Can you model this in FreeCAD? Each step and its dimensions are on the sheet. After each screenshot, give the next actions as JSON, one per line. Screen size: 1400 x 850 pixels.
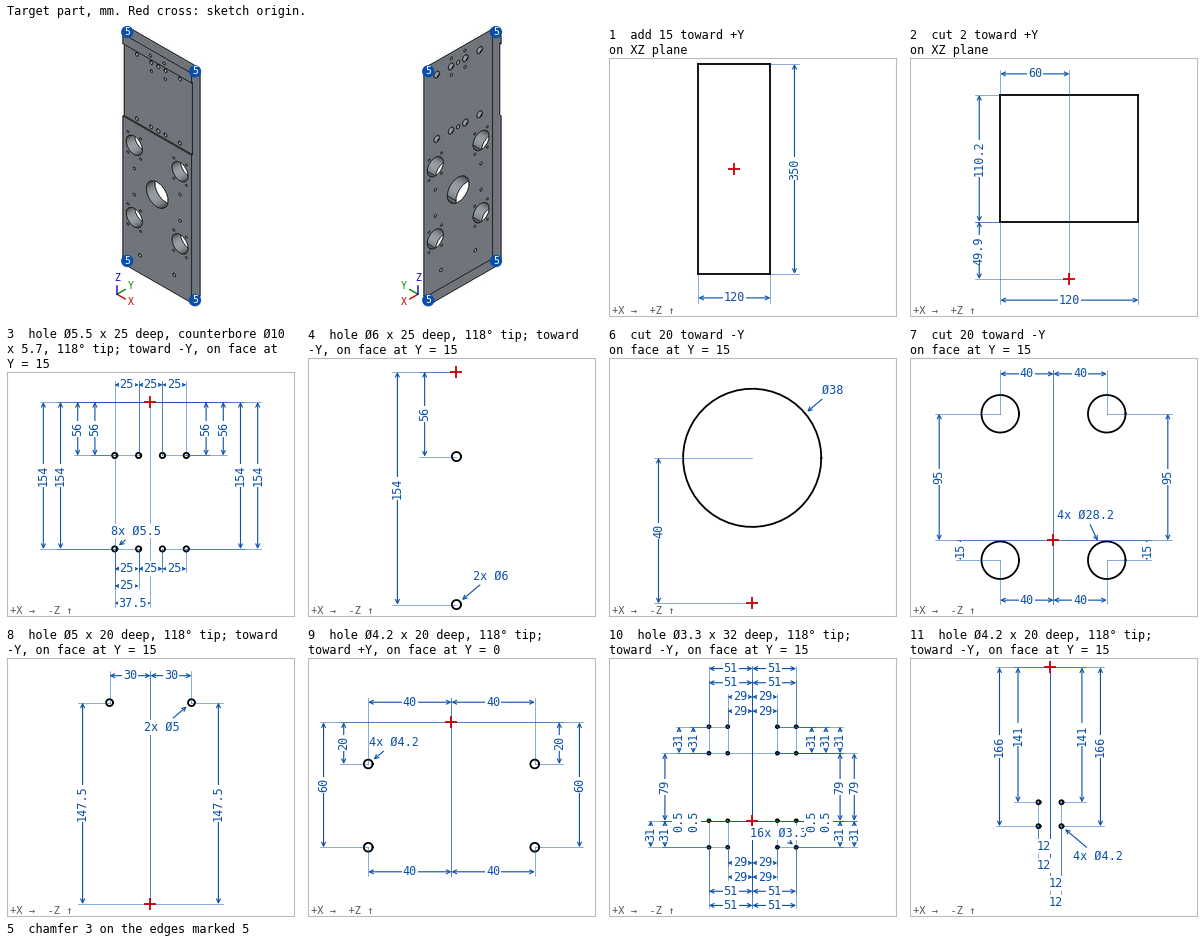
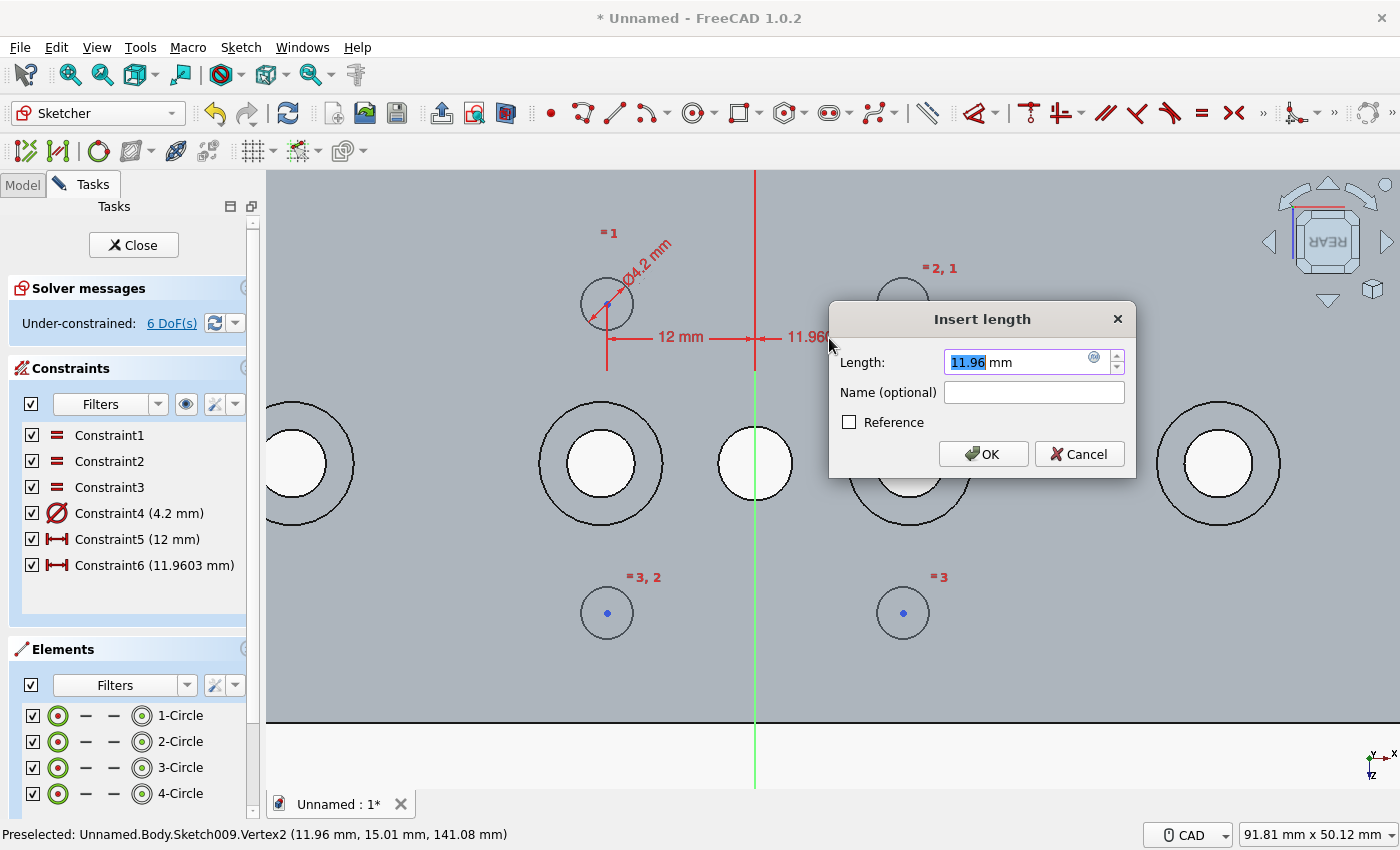
{"action": "type", "text": "12"}
{"action": "key", "text": "Return"}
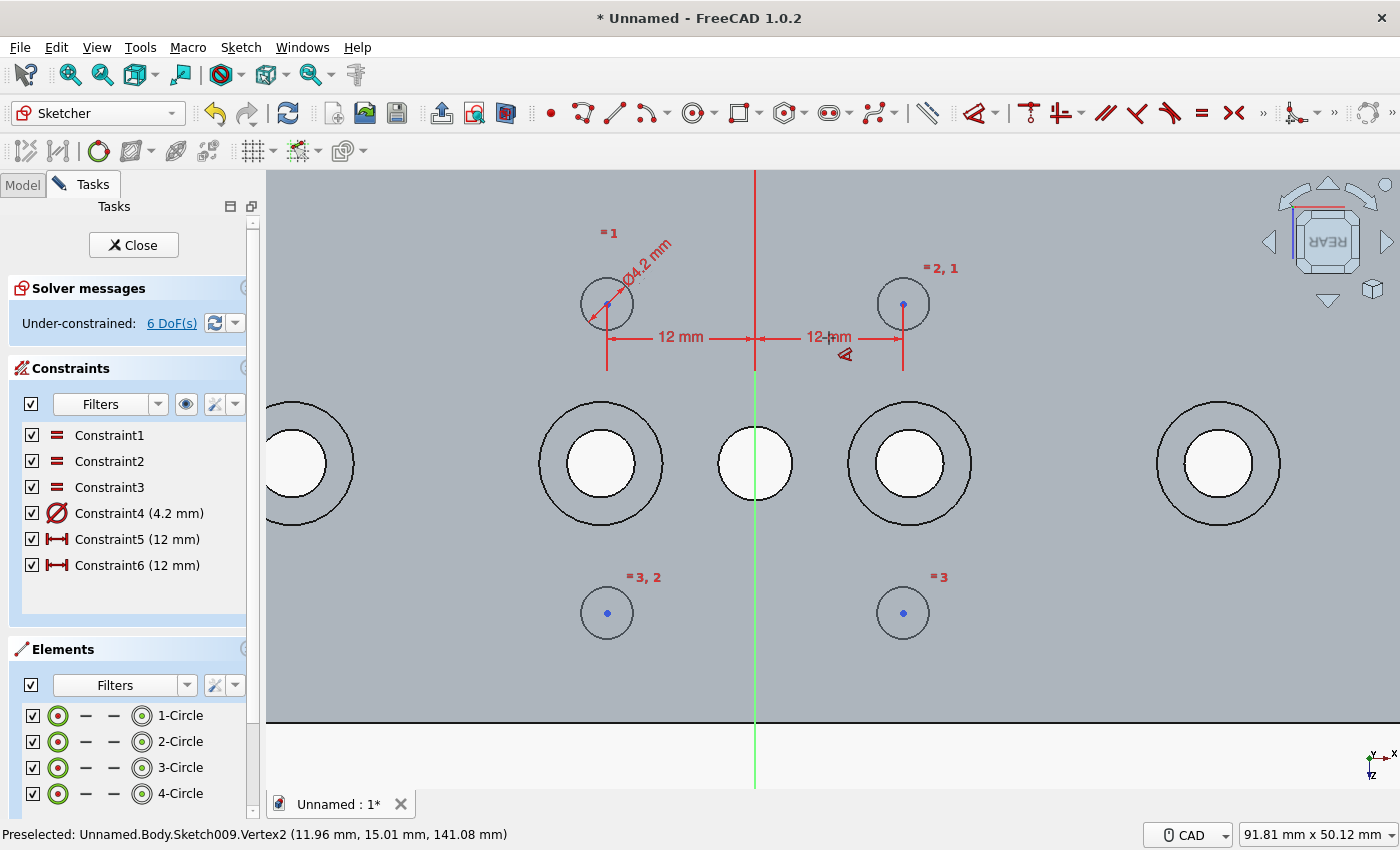
{"action": "left_click", "coordinate": [607, 613]}
{"action": "left_click", "coordinate": [681, 647]}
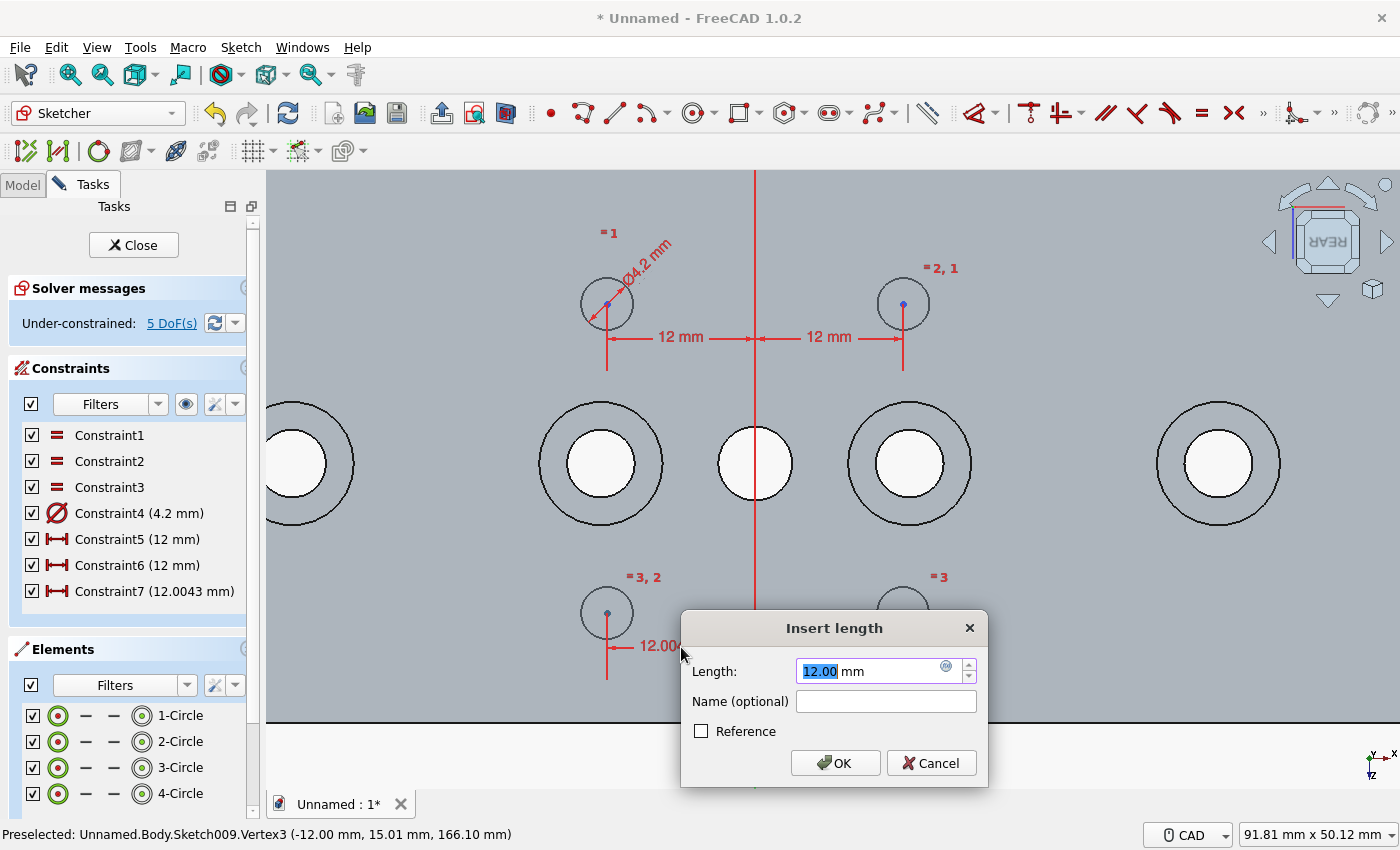
{"action": "type", "text": "12"}
{"action": "key", "text": "Return"}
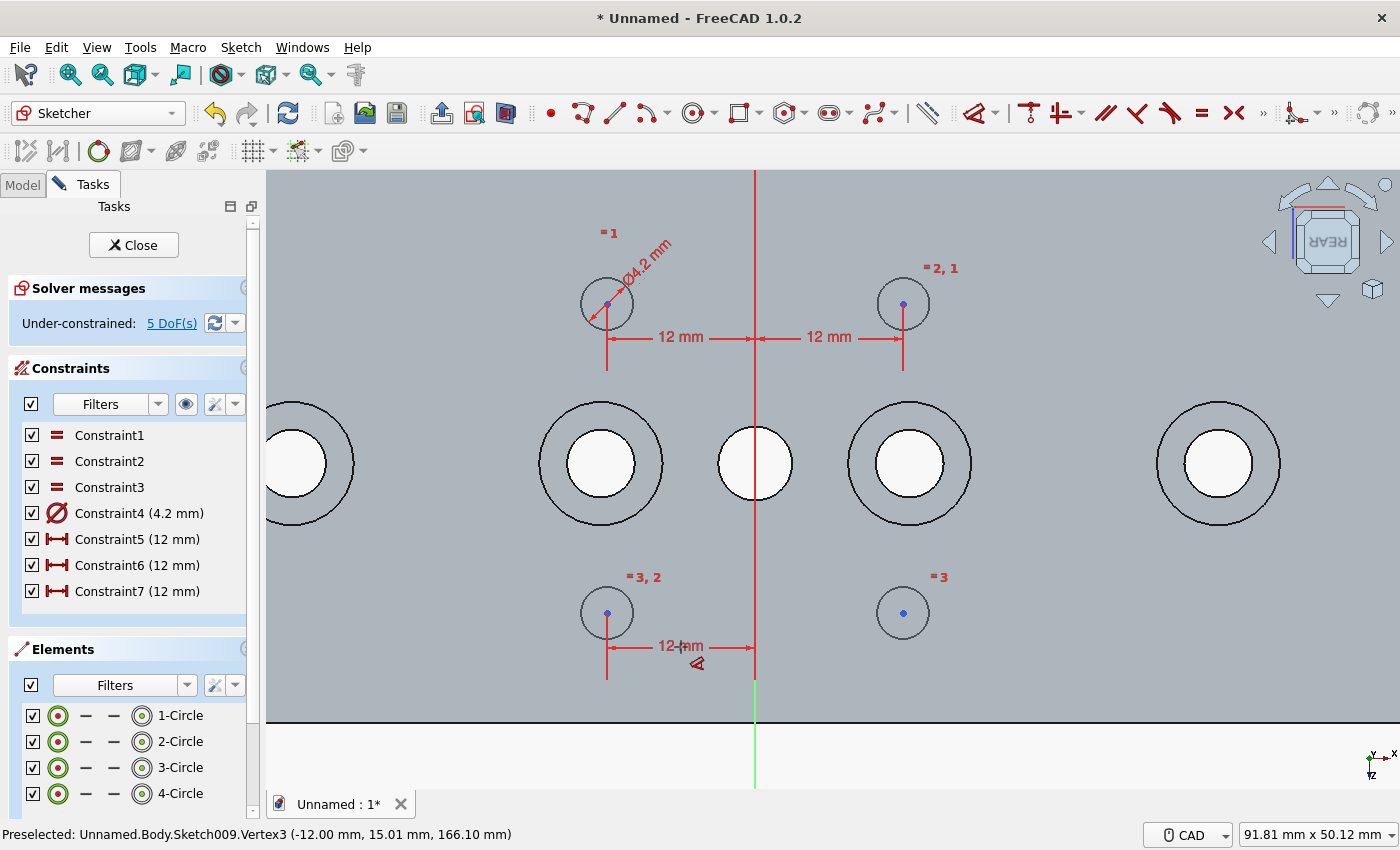
{"action": "left_click", "coordinate": [903, 613]}
{"action": "left_click", "coordinate": [829, 647]}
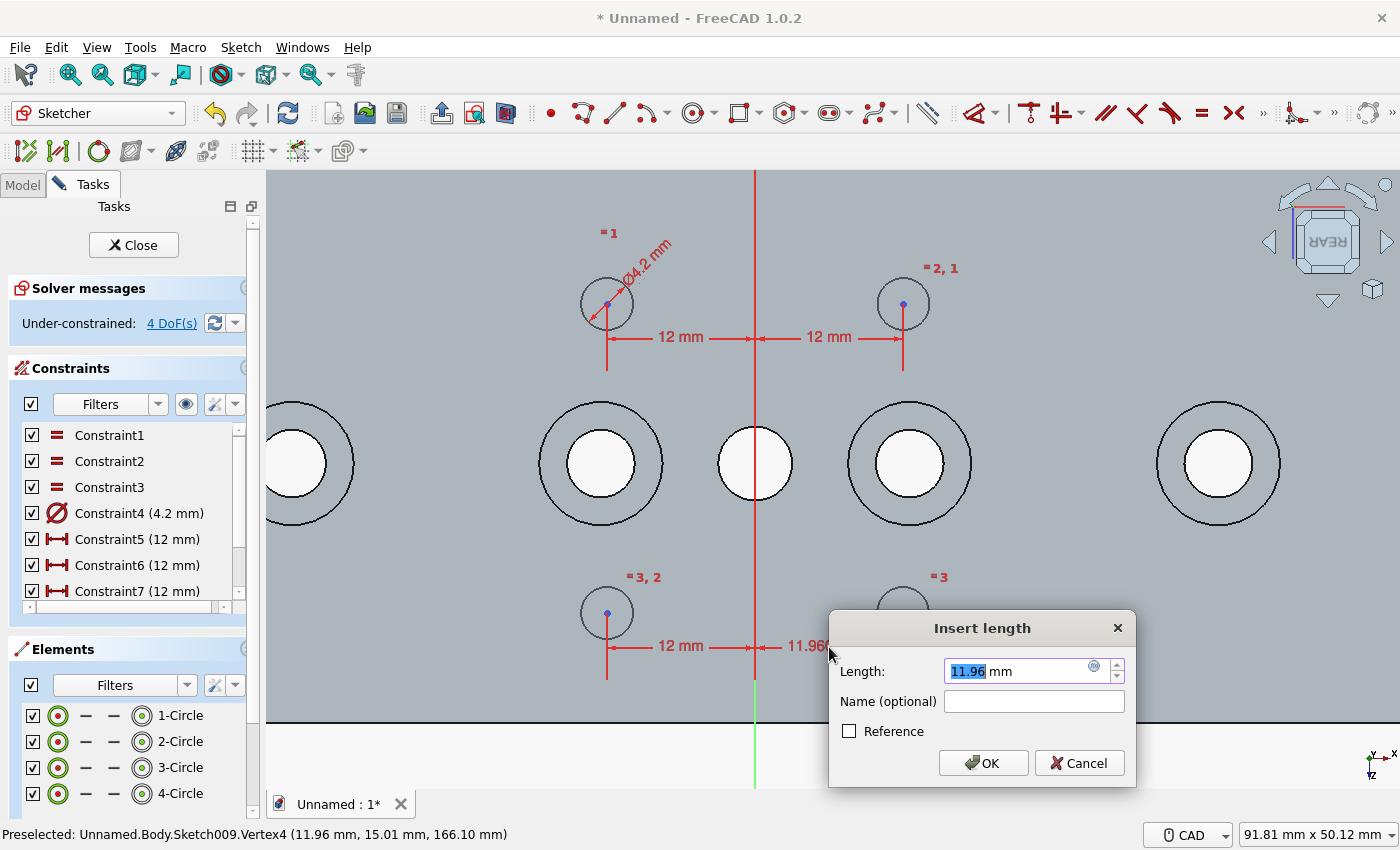
{"action": "type", "text": "12"}
{"action": "key", "text": "Return"}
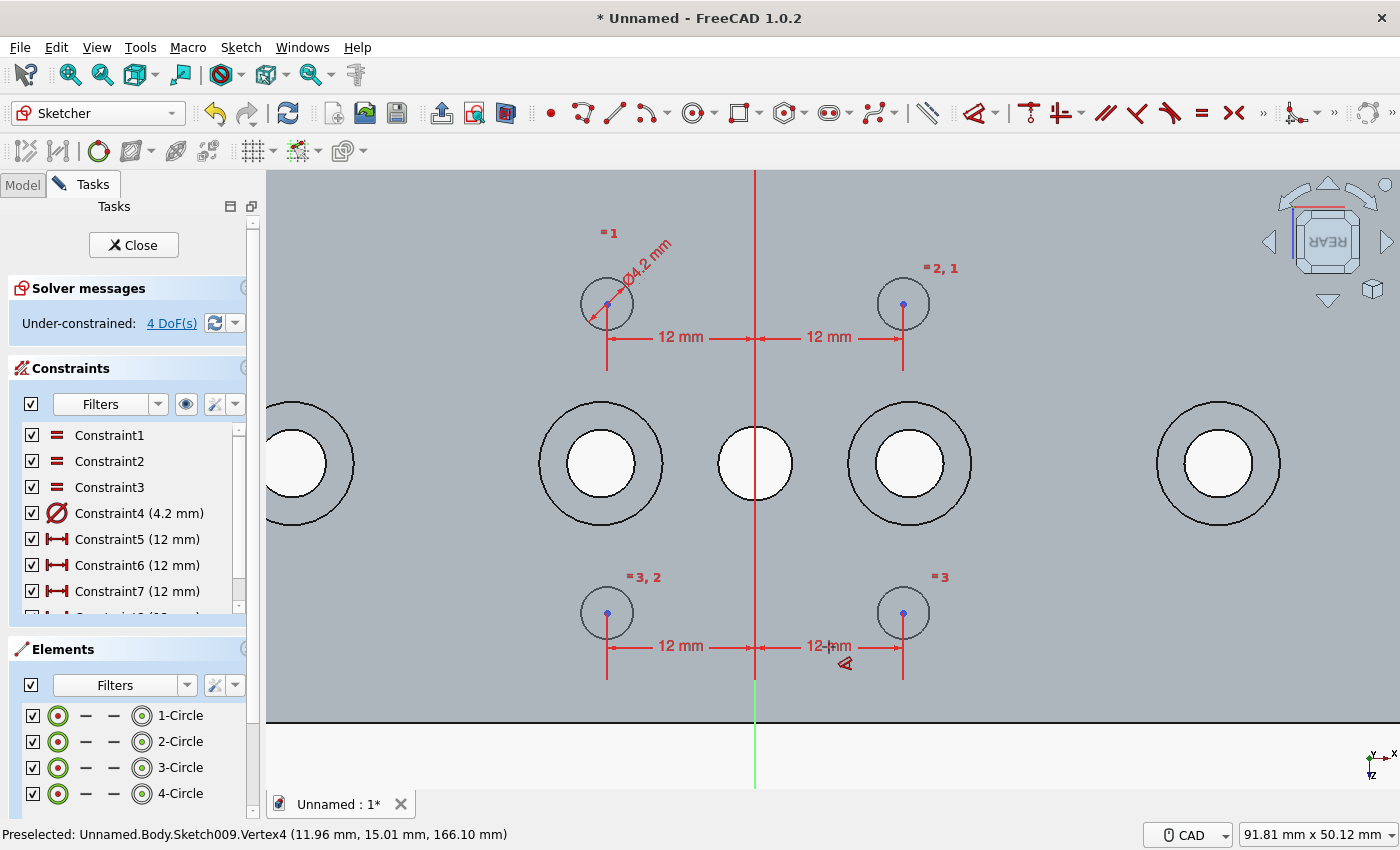
{"action": "left_click", "coordinate": [607, 304]}
{"action": "left_click", "coordinate": [573, 251]}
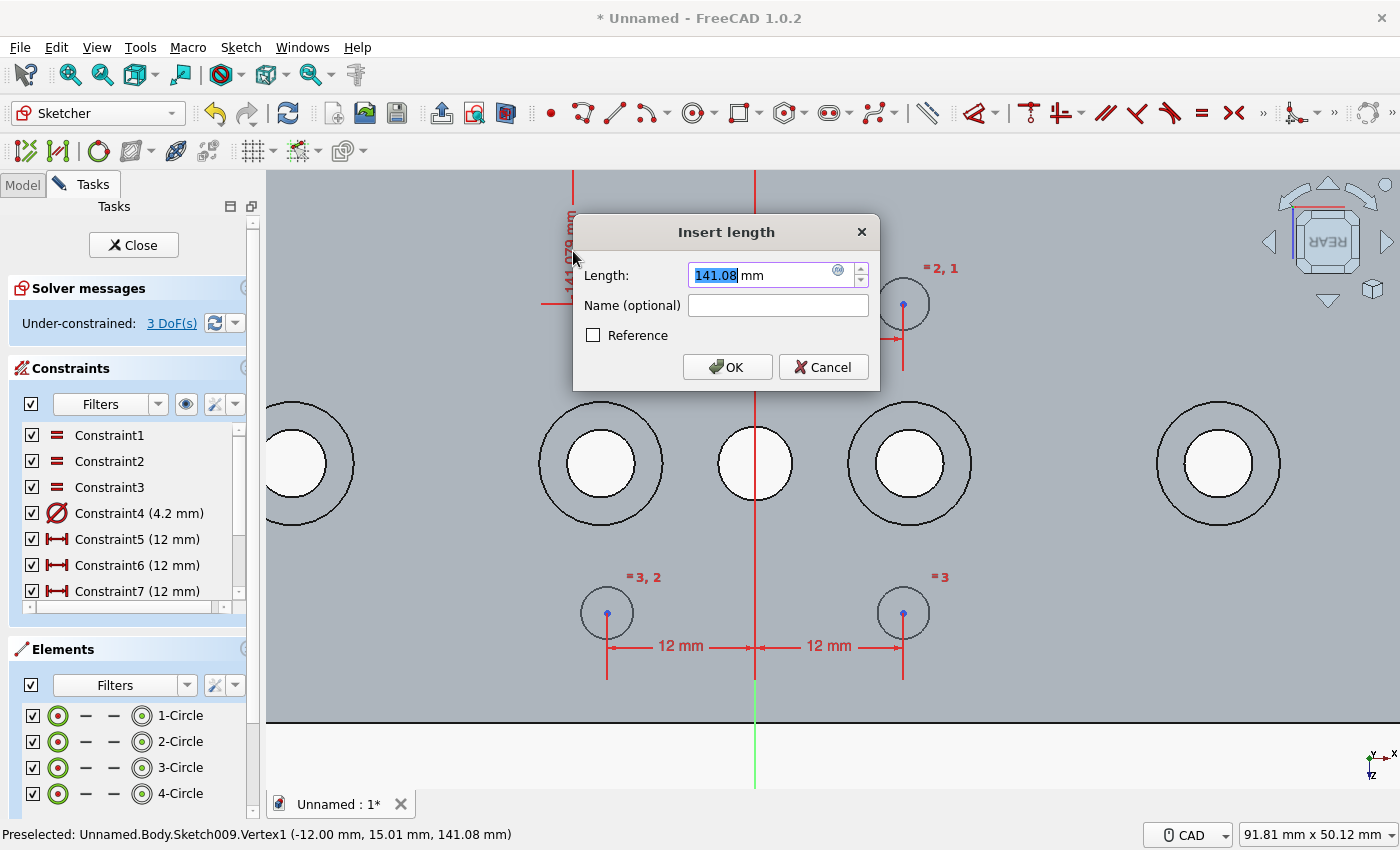
{"action": "type", "text": "141"}
{"action": "key", "text": "Return"}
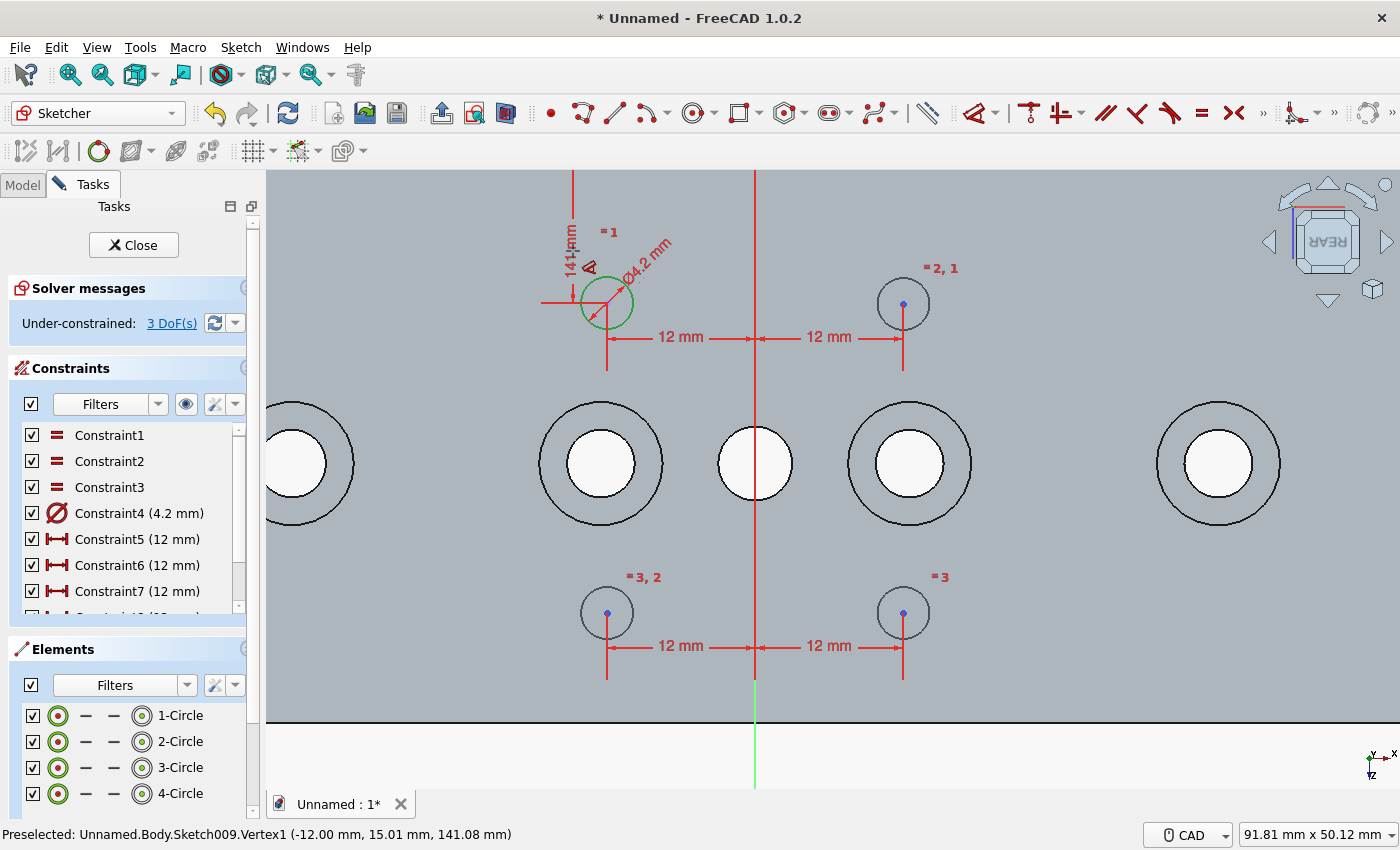
{"action": "left_click", "coordinate": [903, 304]}
{"action": "left_click", "coordinate": [937, 251]}